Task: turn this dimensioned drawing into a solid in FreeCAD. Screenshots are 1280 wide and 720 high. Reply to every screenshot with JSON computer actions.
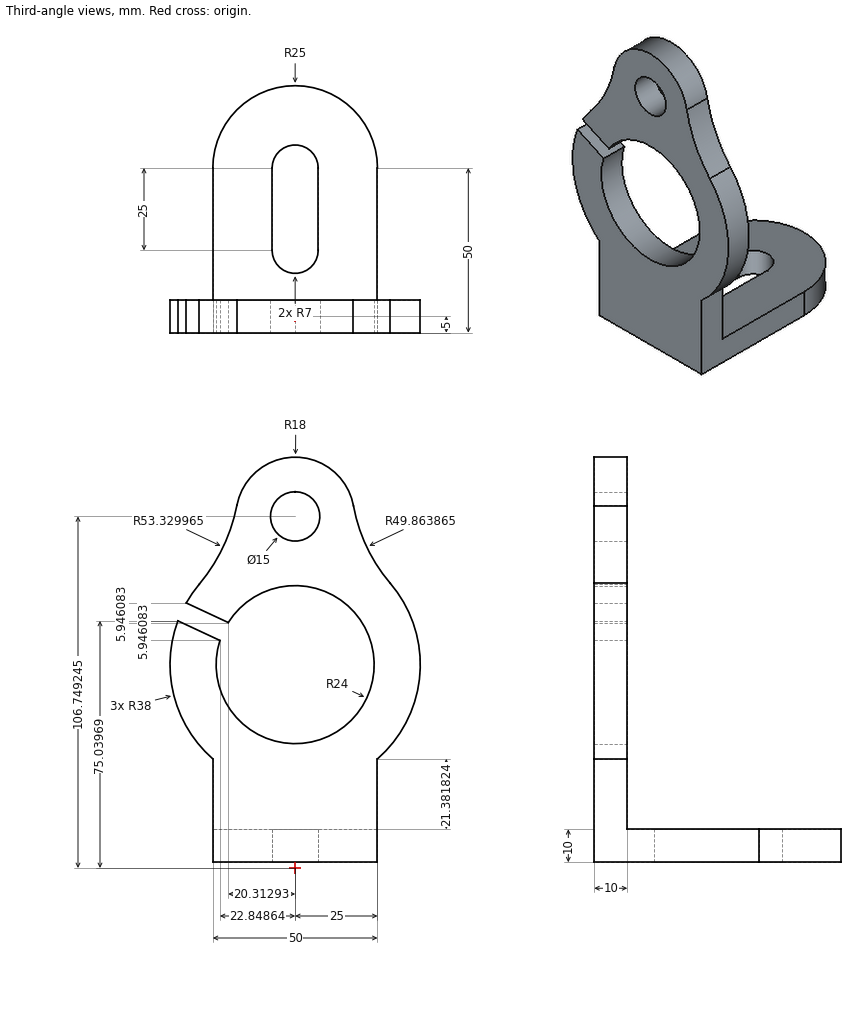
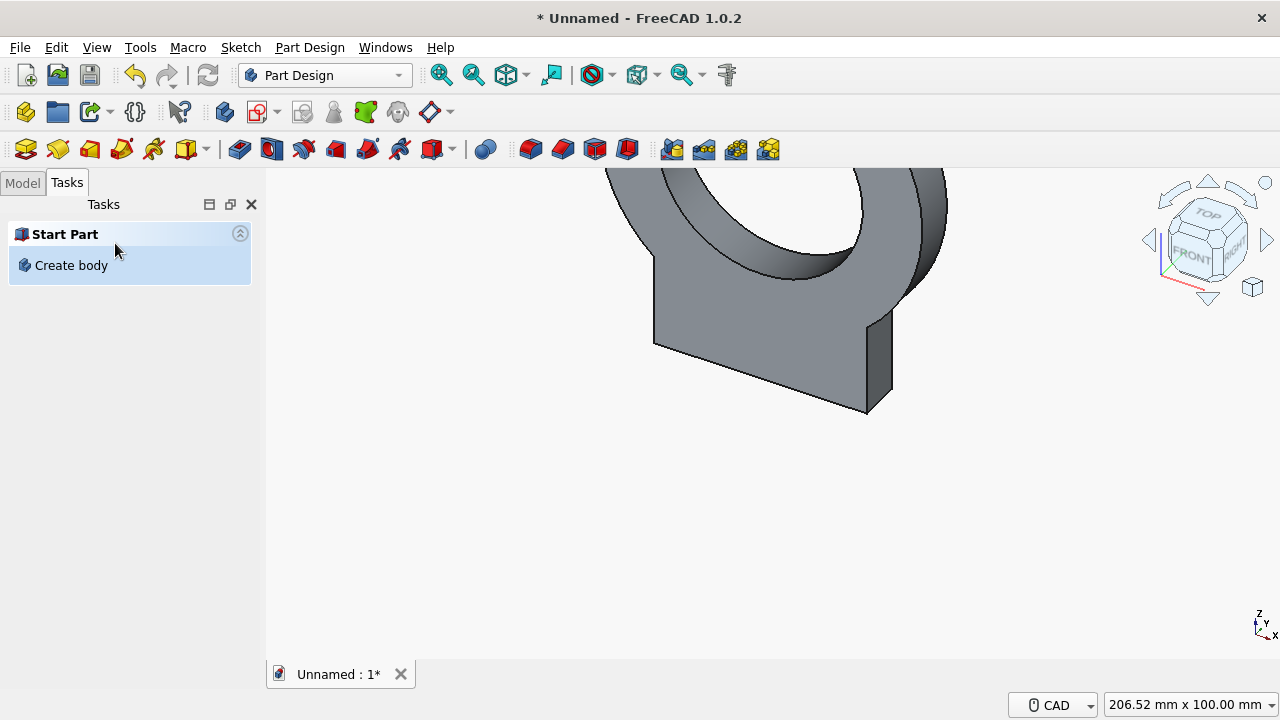
{"action": "left_click", "coordinate": [442, 76]}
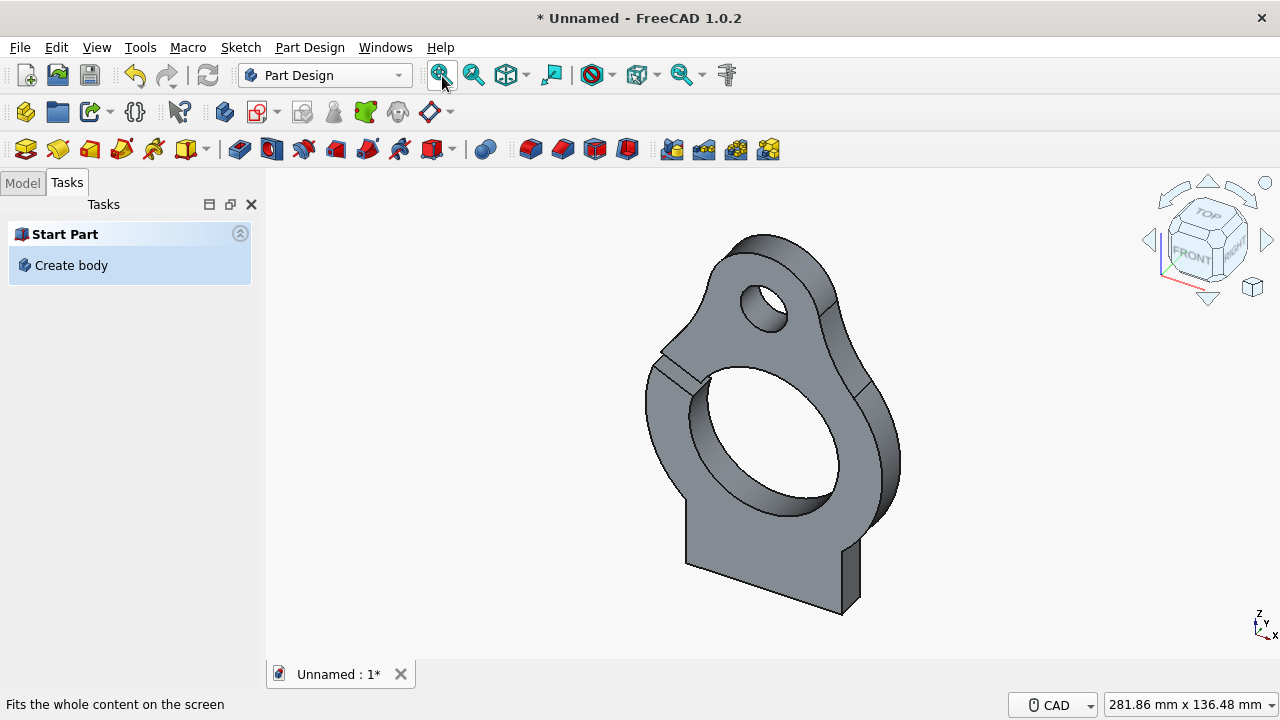
{"action": "key", "text": "5"}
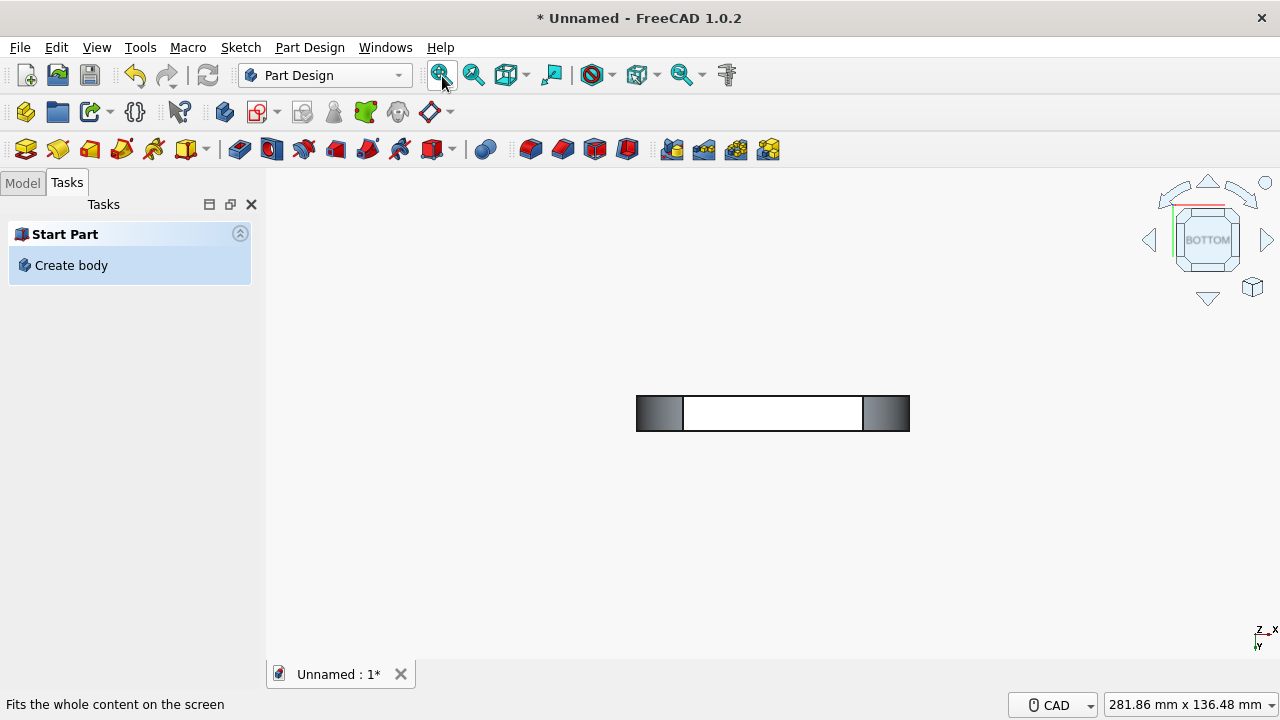
{"action": "left_click", "coordinate": [442, 76]}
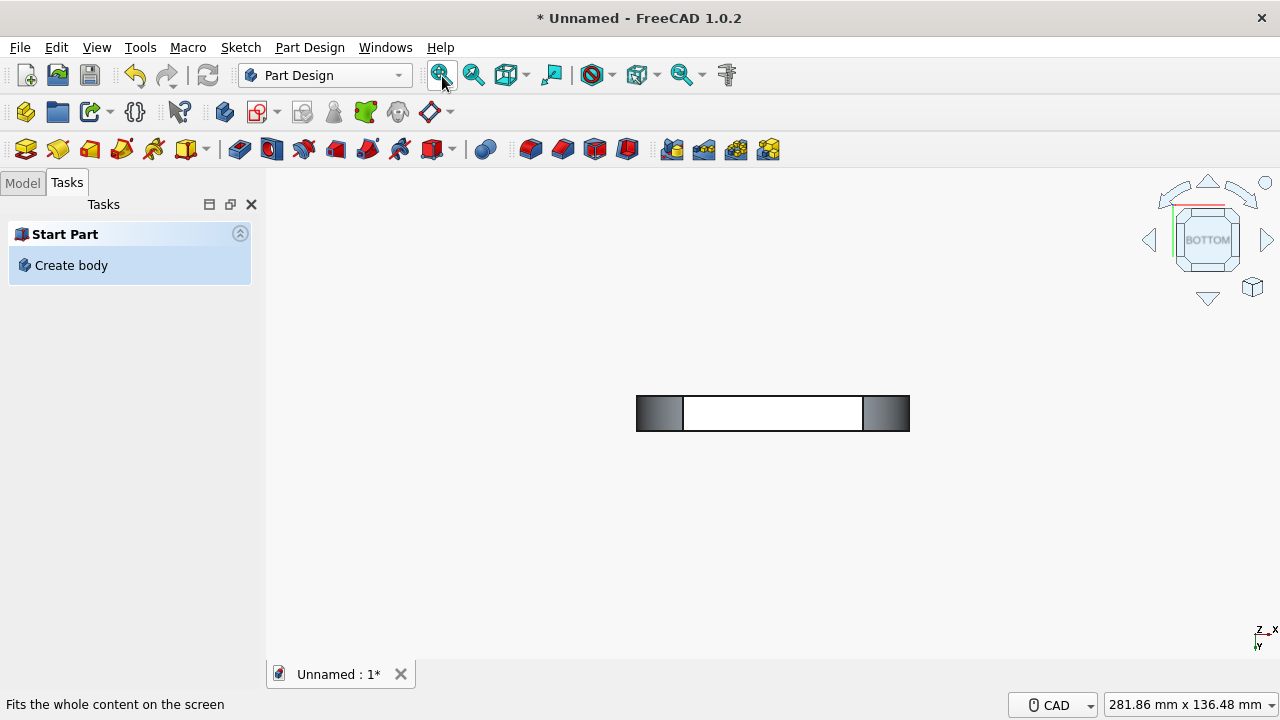
{"action": "left_click", "coordinate": [824, 413]}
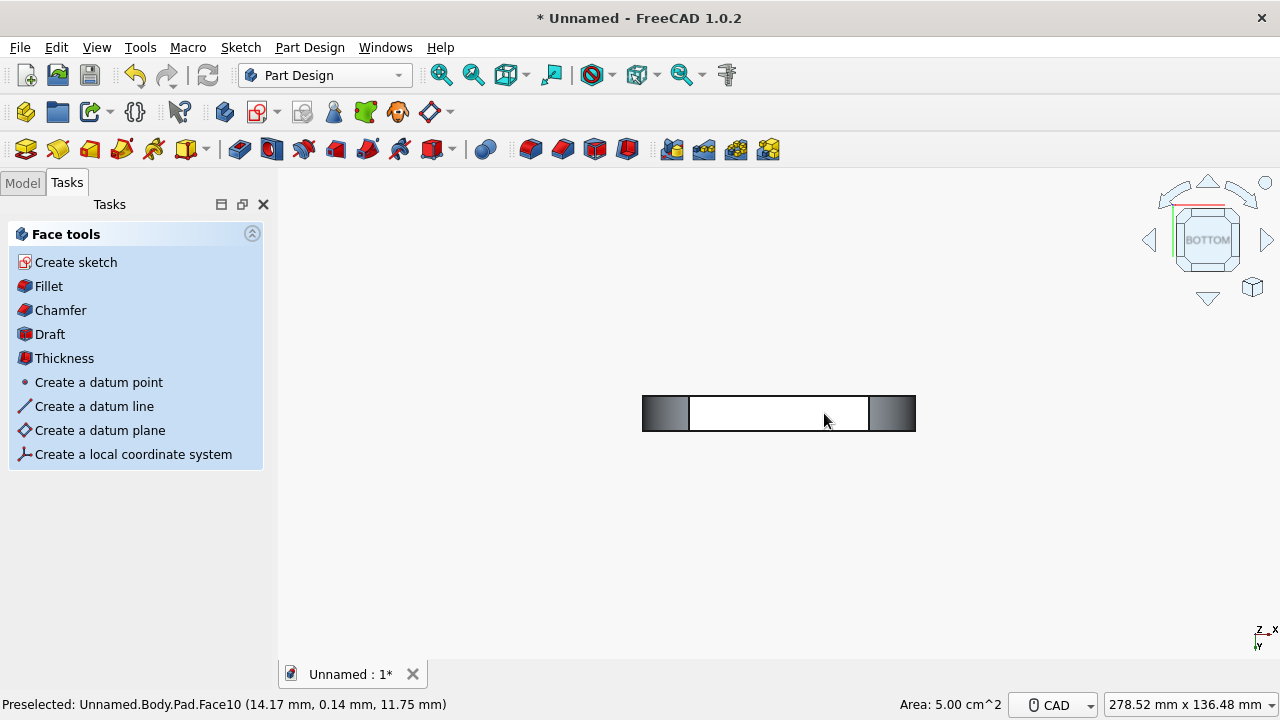
{"action": "left_click", "coordinate": [258, 112]}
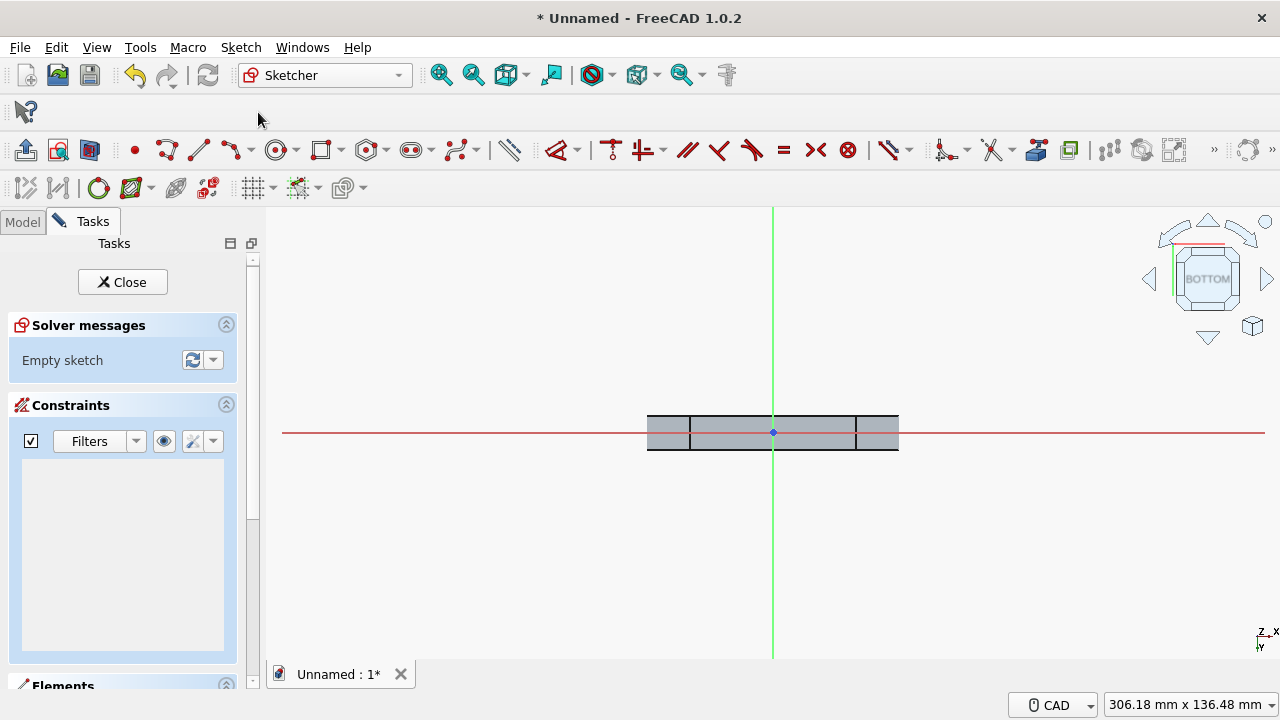
{"action": "scroll", "coordinate": [395, 235], "scroll_direction": "down", "scroll_amount": 1}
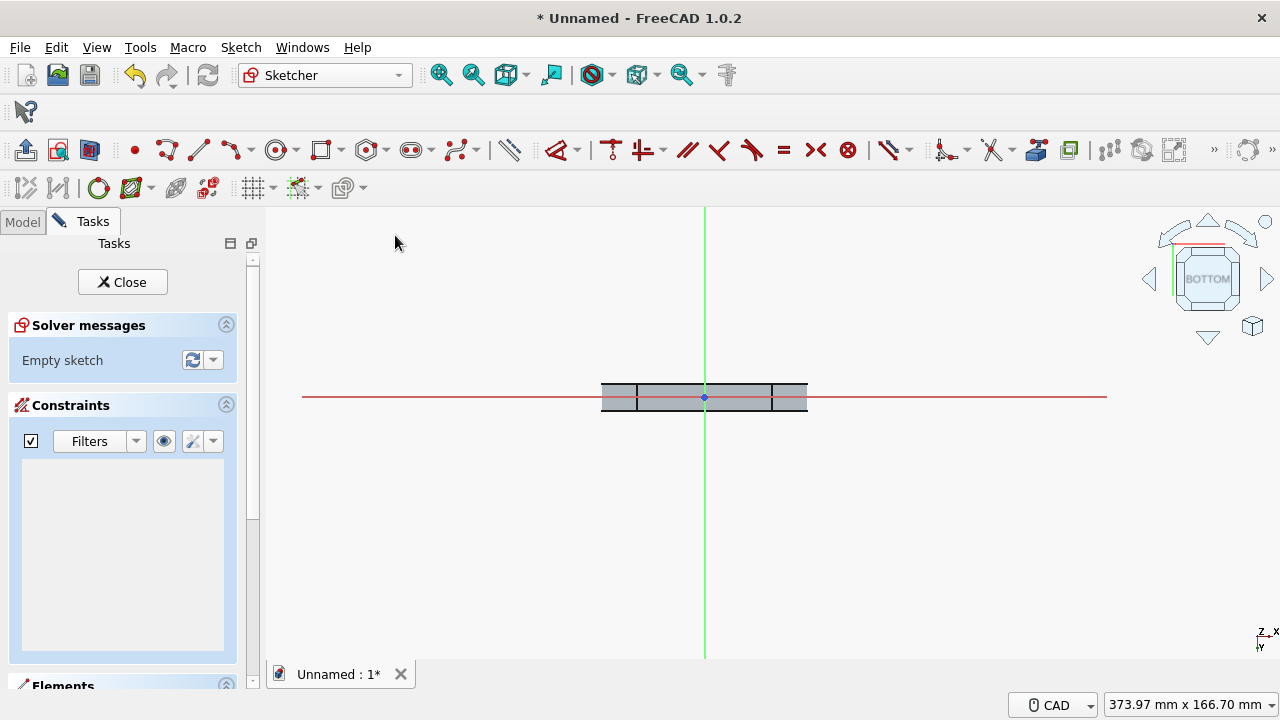
{"action": "scroll", "coordinate": [705, 591], "scroll_direction": "up", "scroll_amount": 2}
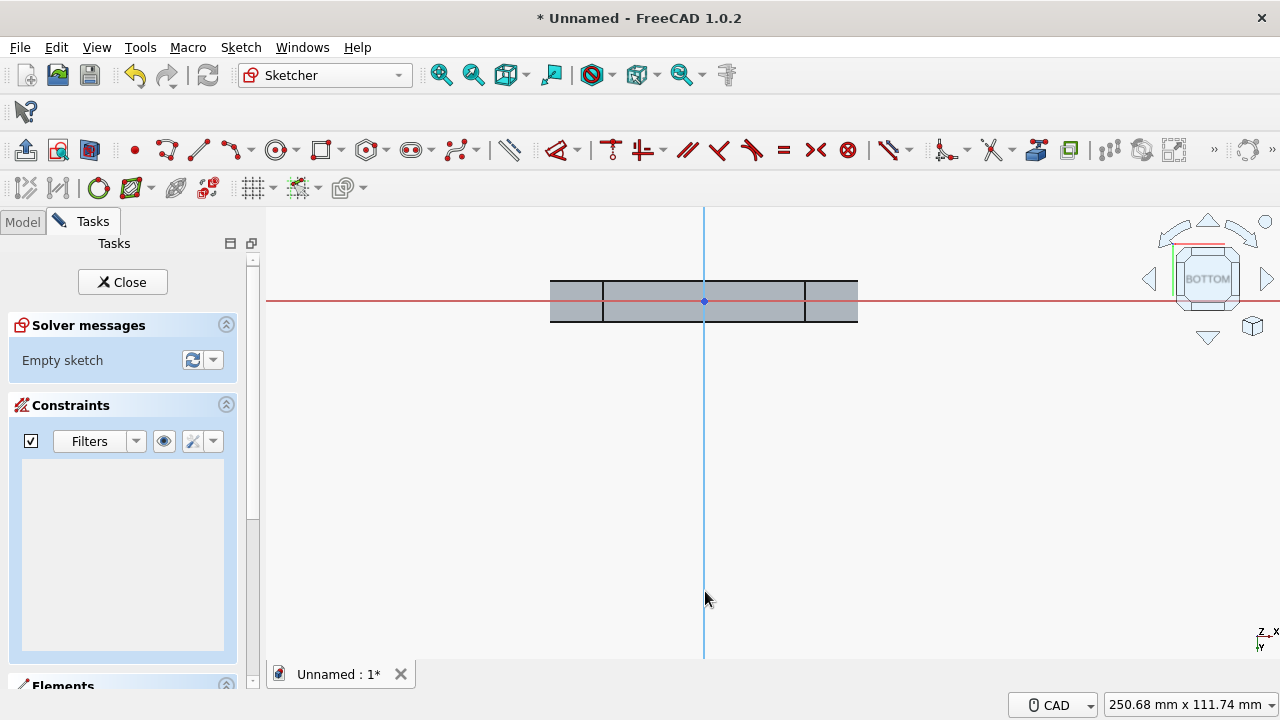
{"action": "left_click", "coordinate": [168, 150]}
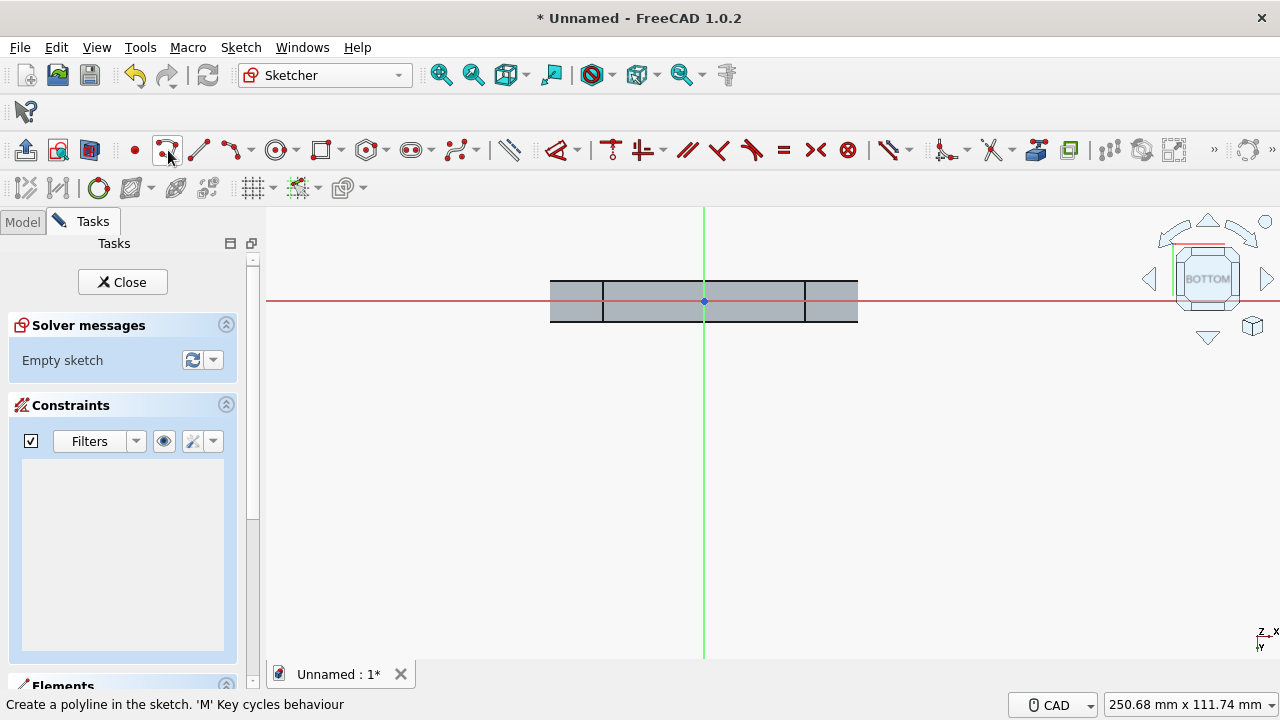
{"action": "left_click", "coordinate": [805, 483]}
{"action": "left_click", "coordinate": [805, 281]}
{"action": "left_click", "coordinate": [603, 281]}
{"action": "left_click", "coordinate": [603, 483]}
{"action": "right_click", "coordinate": [603, 483]}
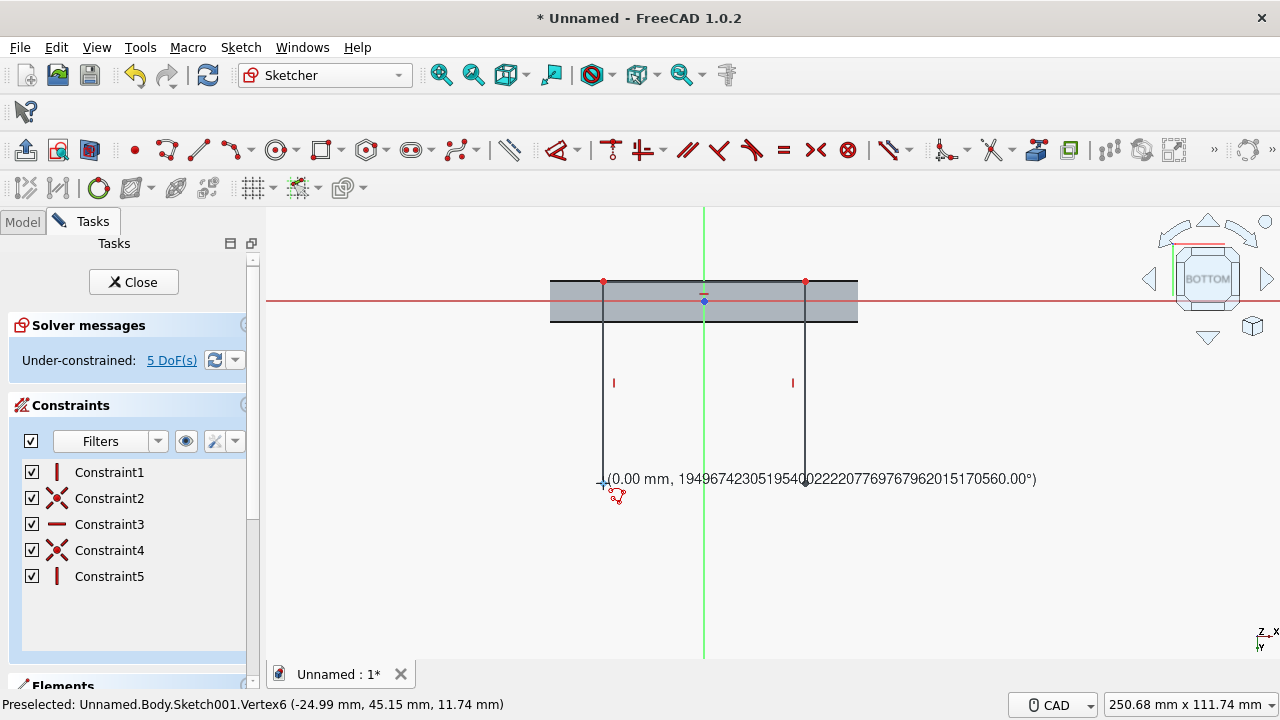
{"action": "left_click", "coordinate": [232, 150]}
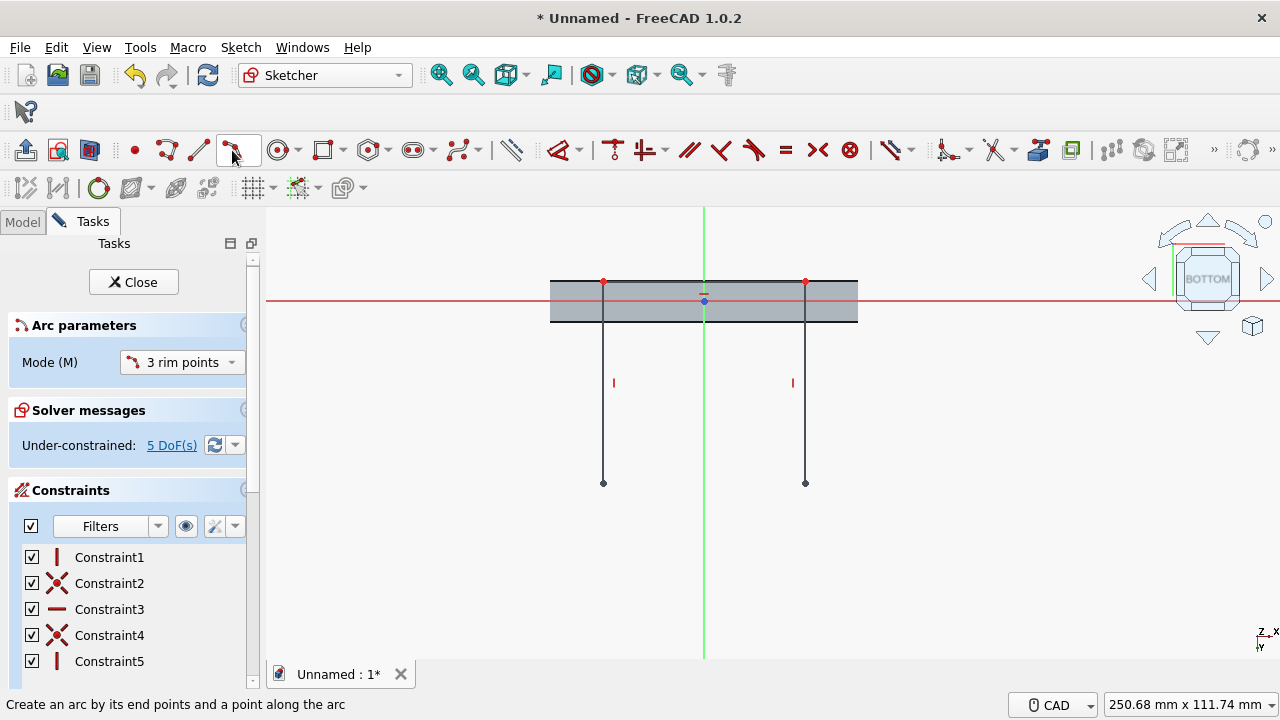
{"action": "left_click", "coordinate": [603, 484]}
{"action": "left_click", "coordinate": [805, 484]}
{"action": "left_click", "coordinate": [673, 580]}